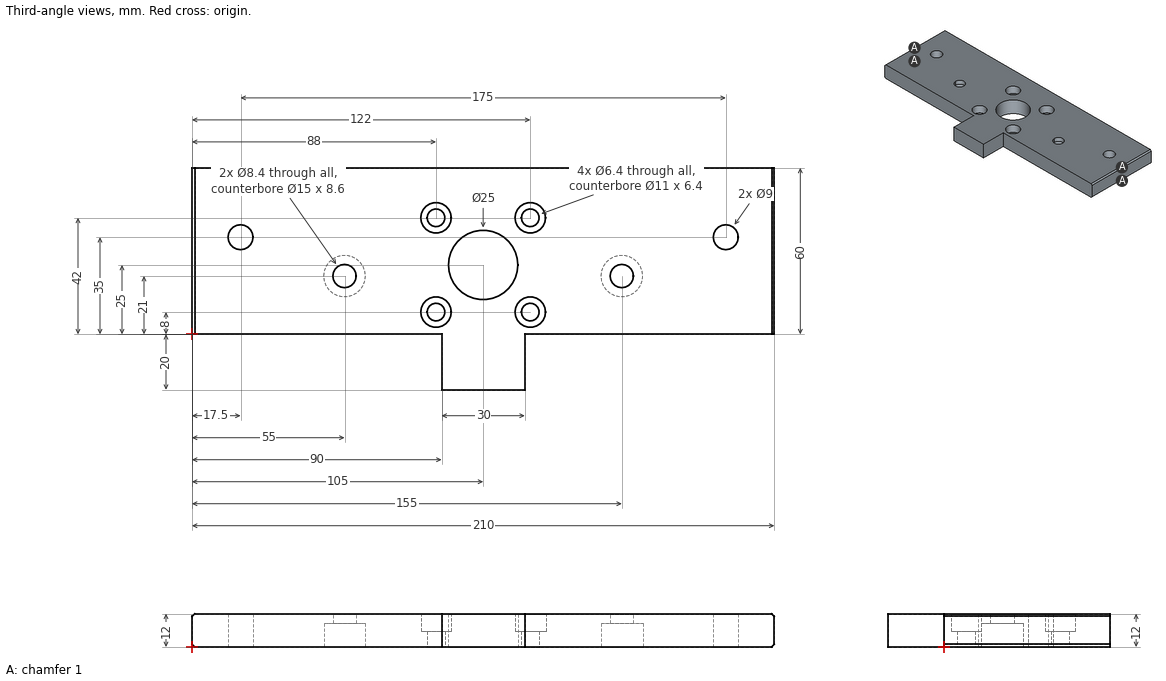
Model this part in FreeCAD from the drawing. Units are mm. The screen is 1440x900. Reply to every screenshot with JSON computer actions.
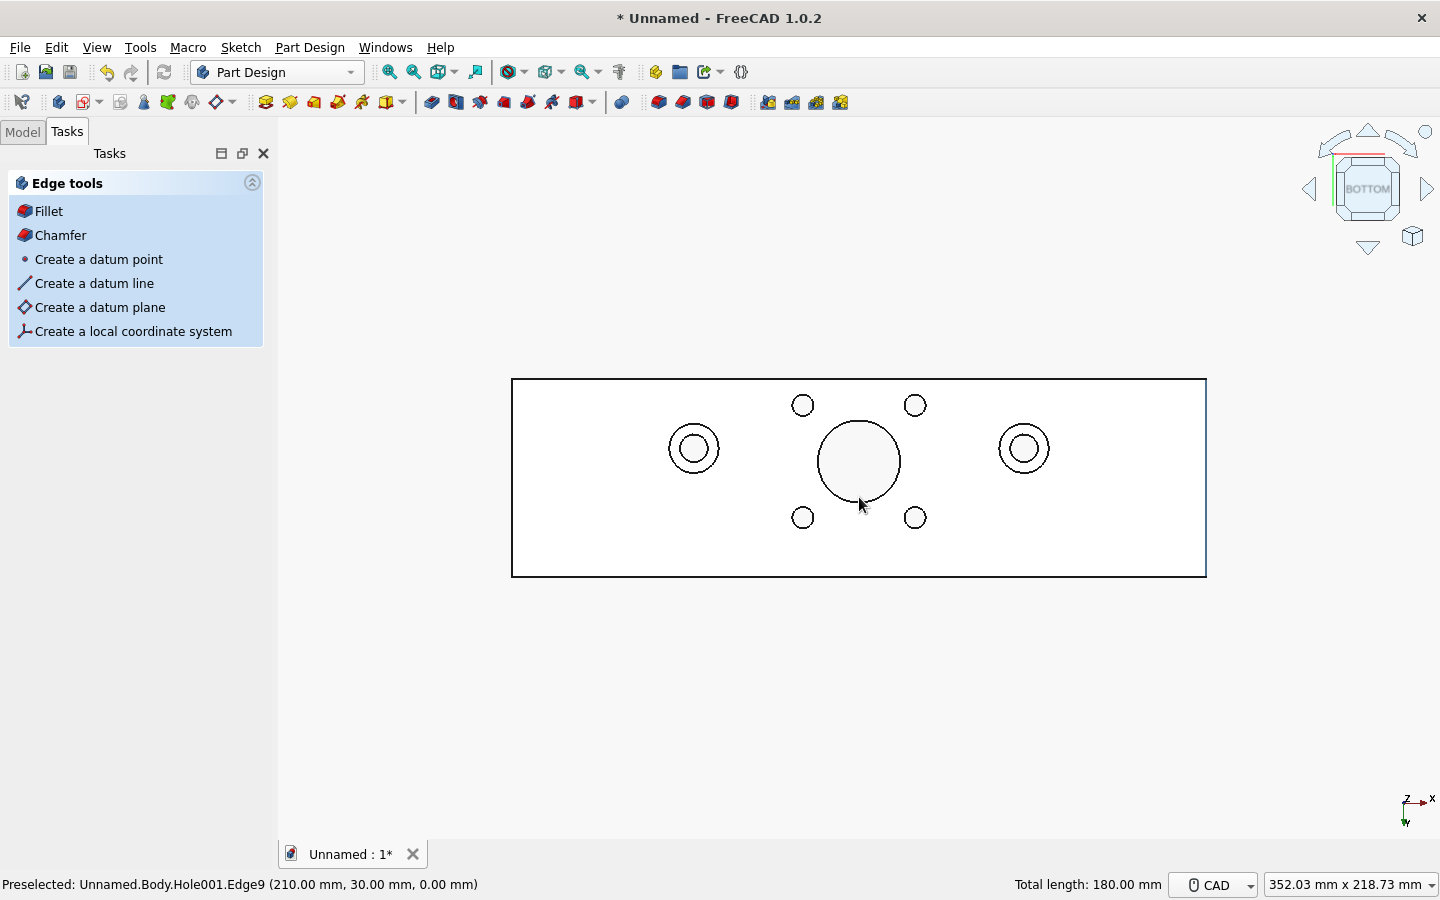
{"action": "left_click", "coordinate": [512, 477], "text": "ctrl"}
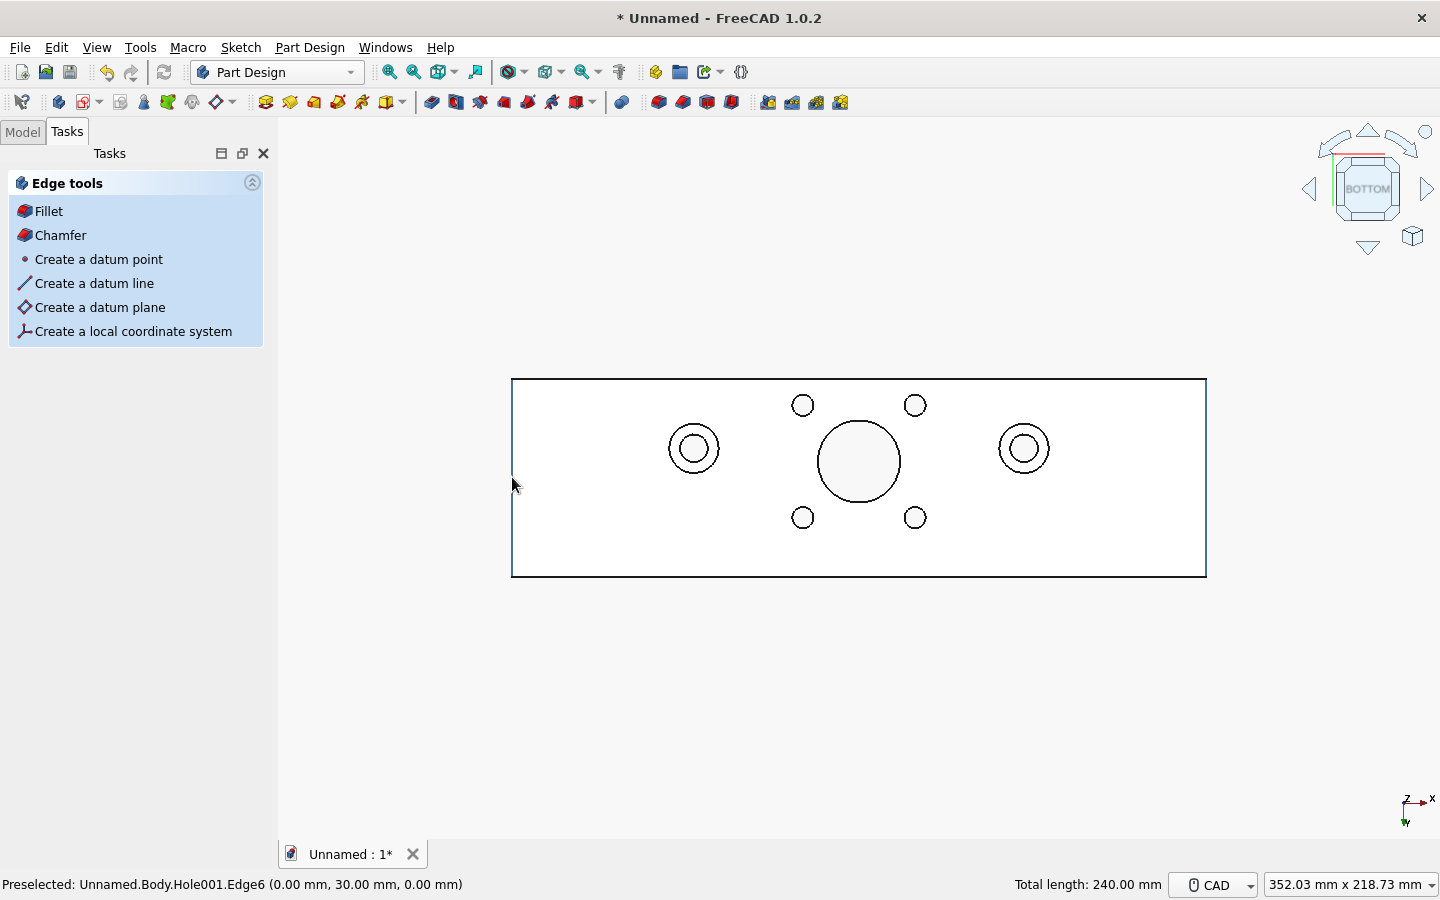
{"action": "left_click", "coordinate": [684, 102]}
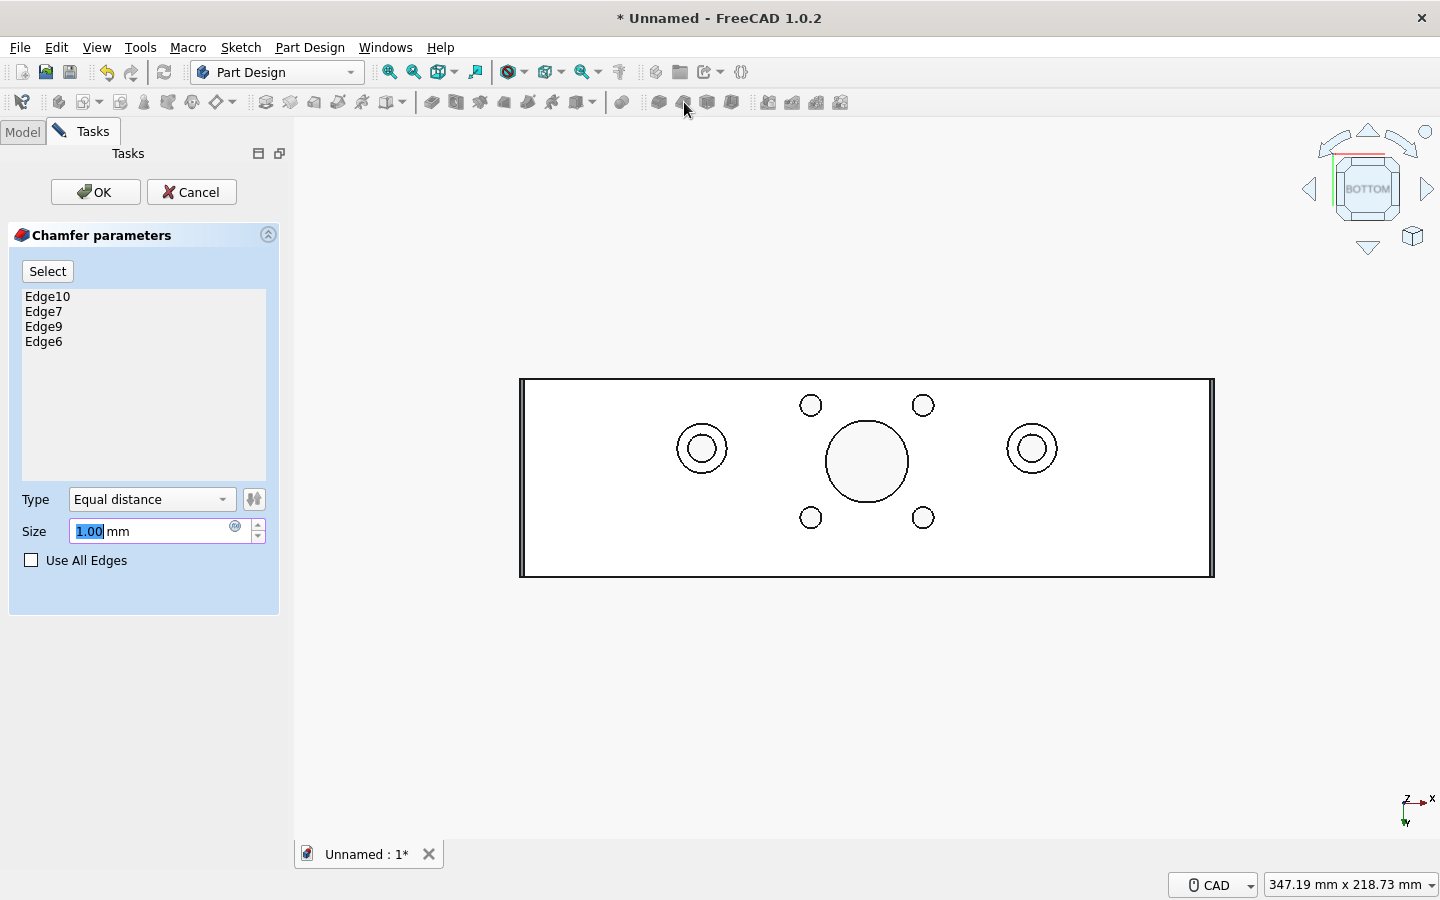
{"action": "type", "text": "1"}
{"action": "key", "text": "Tab"}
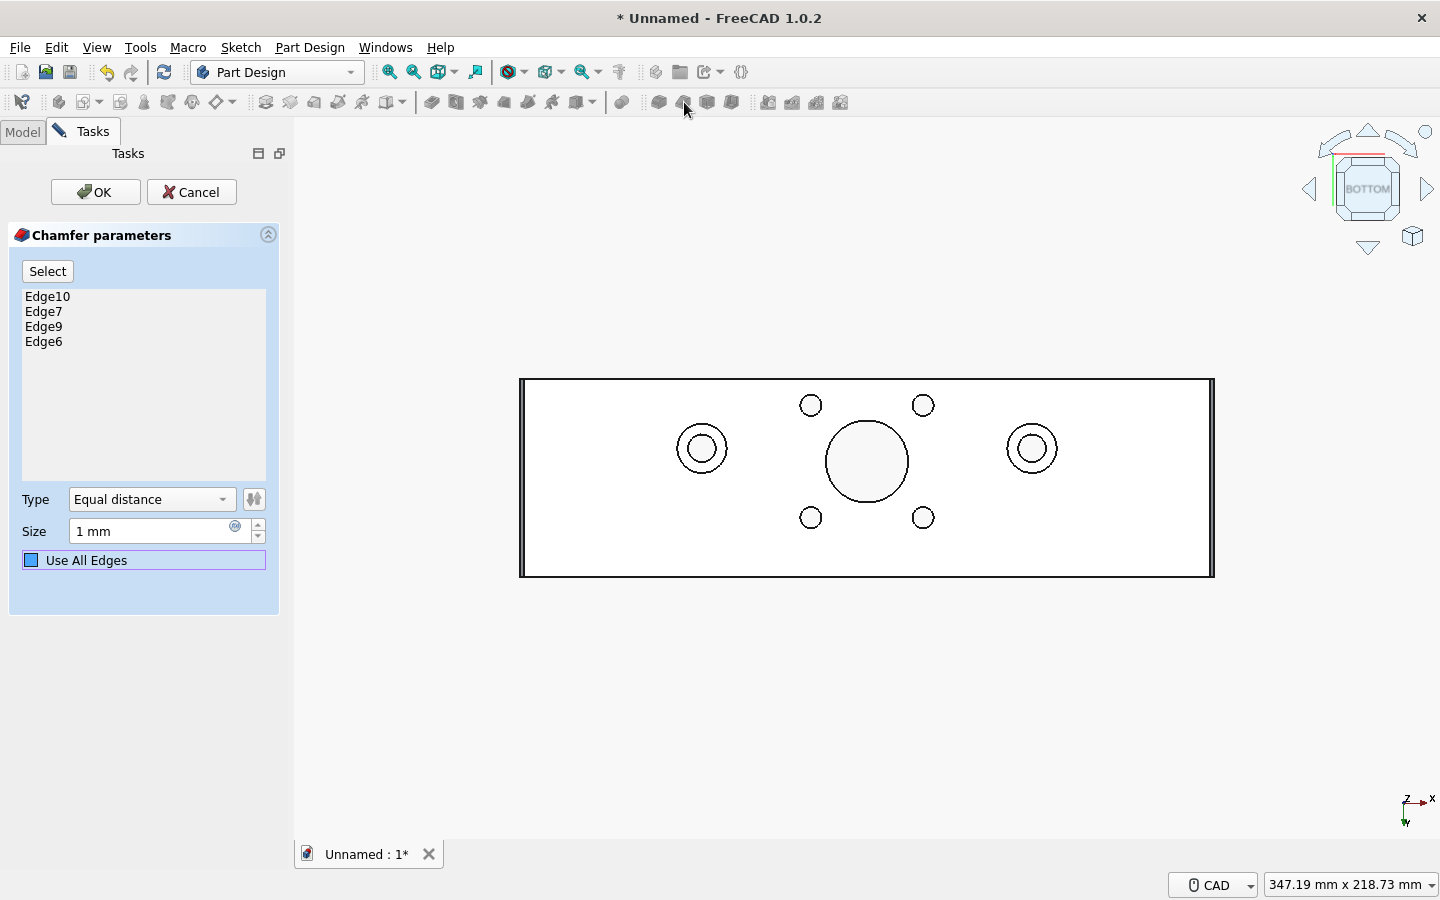
{"action": "left_click", "coordinate": [96, 192]}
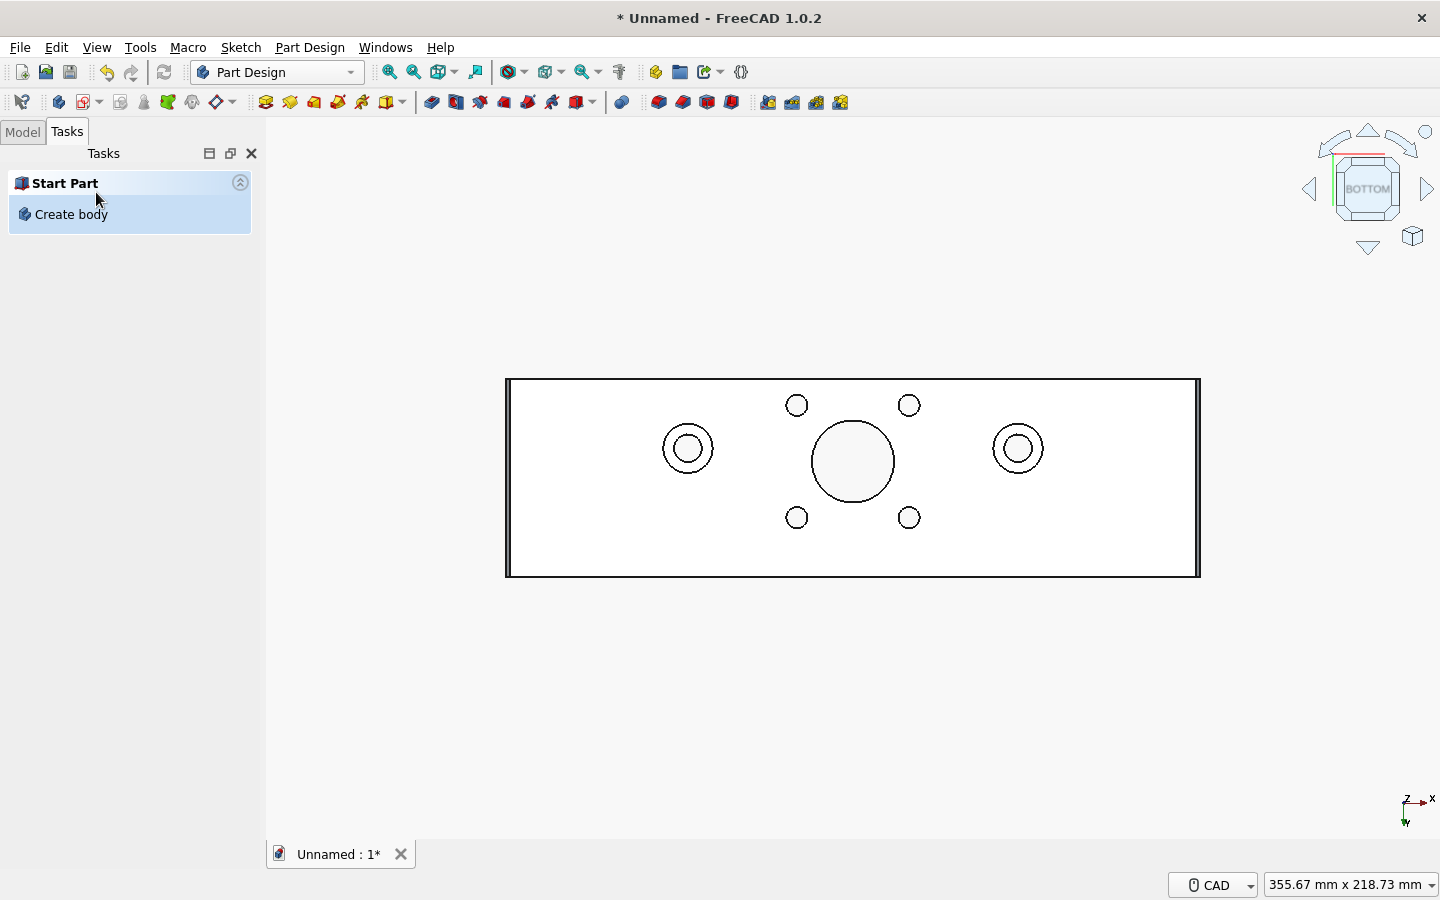
{"action": "left_click", "coordinate": [1147, 505]}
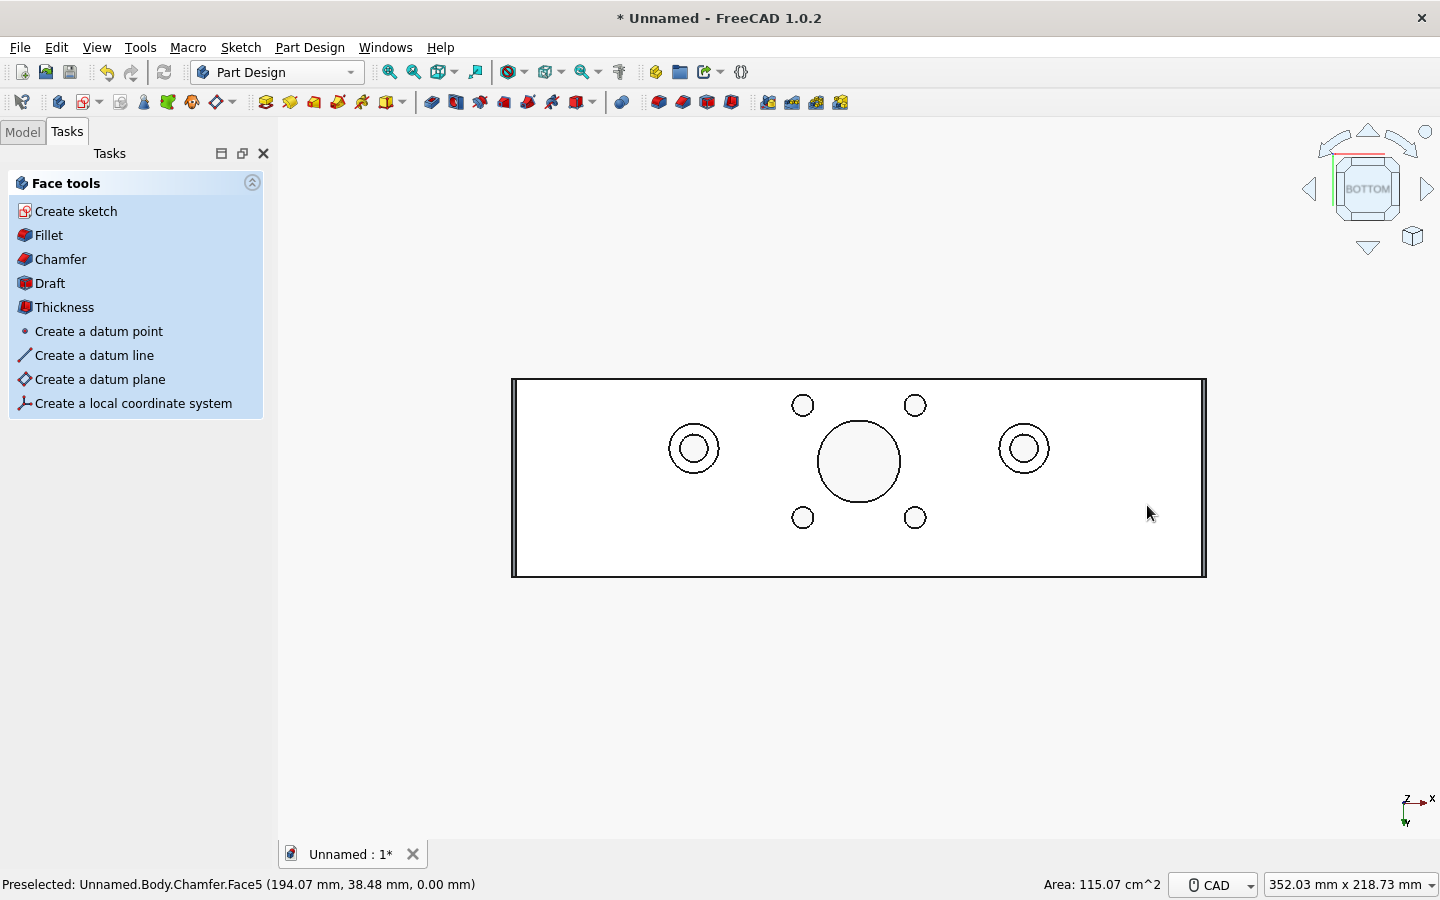
{"action": "left_click", "coordinate": [84, 102]}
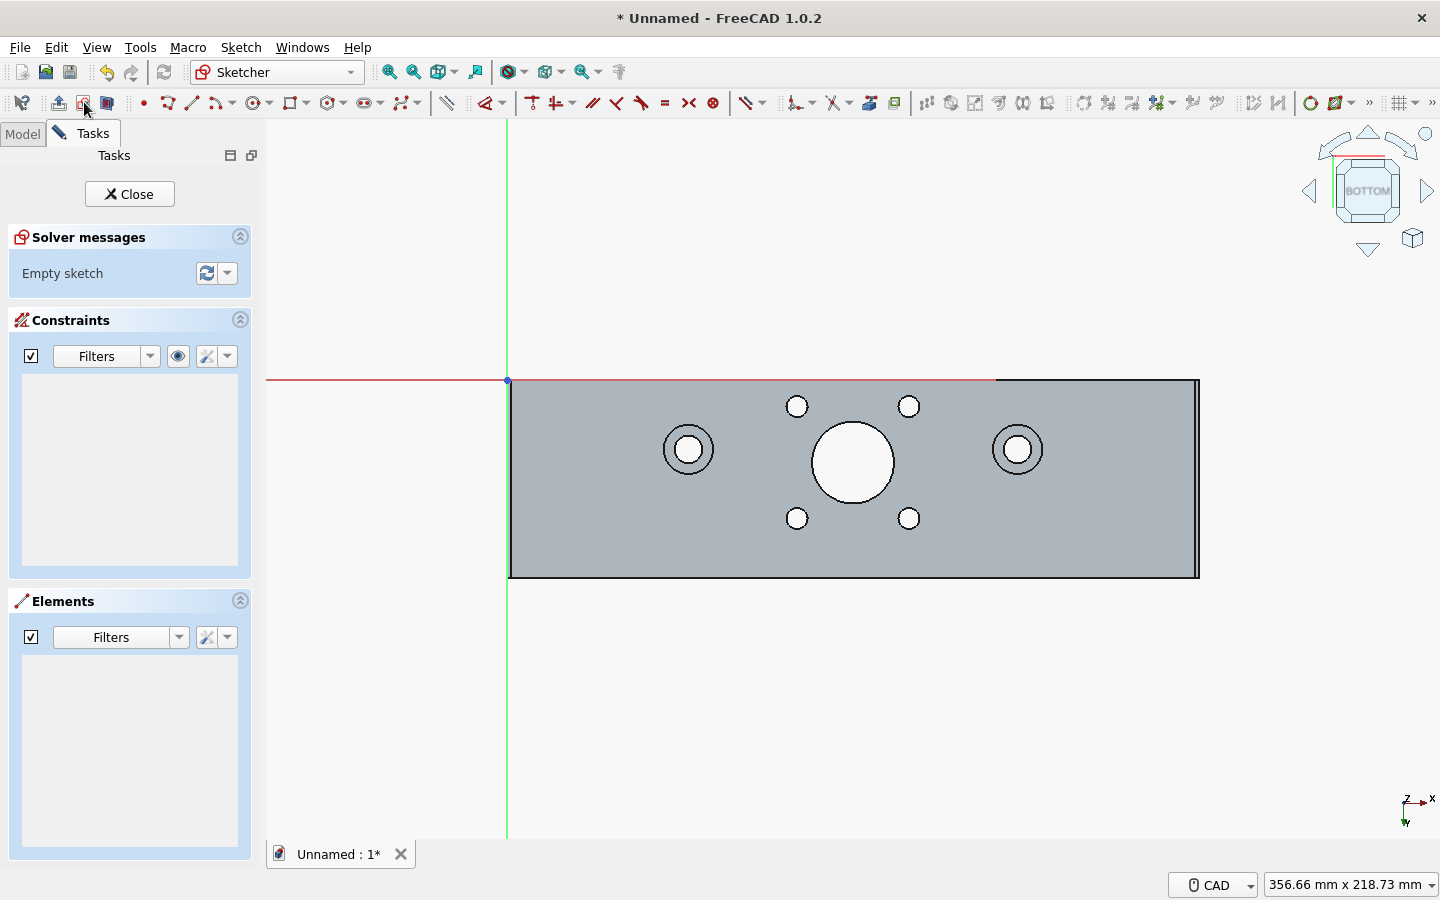
{"action": "key", "text": "g c"}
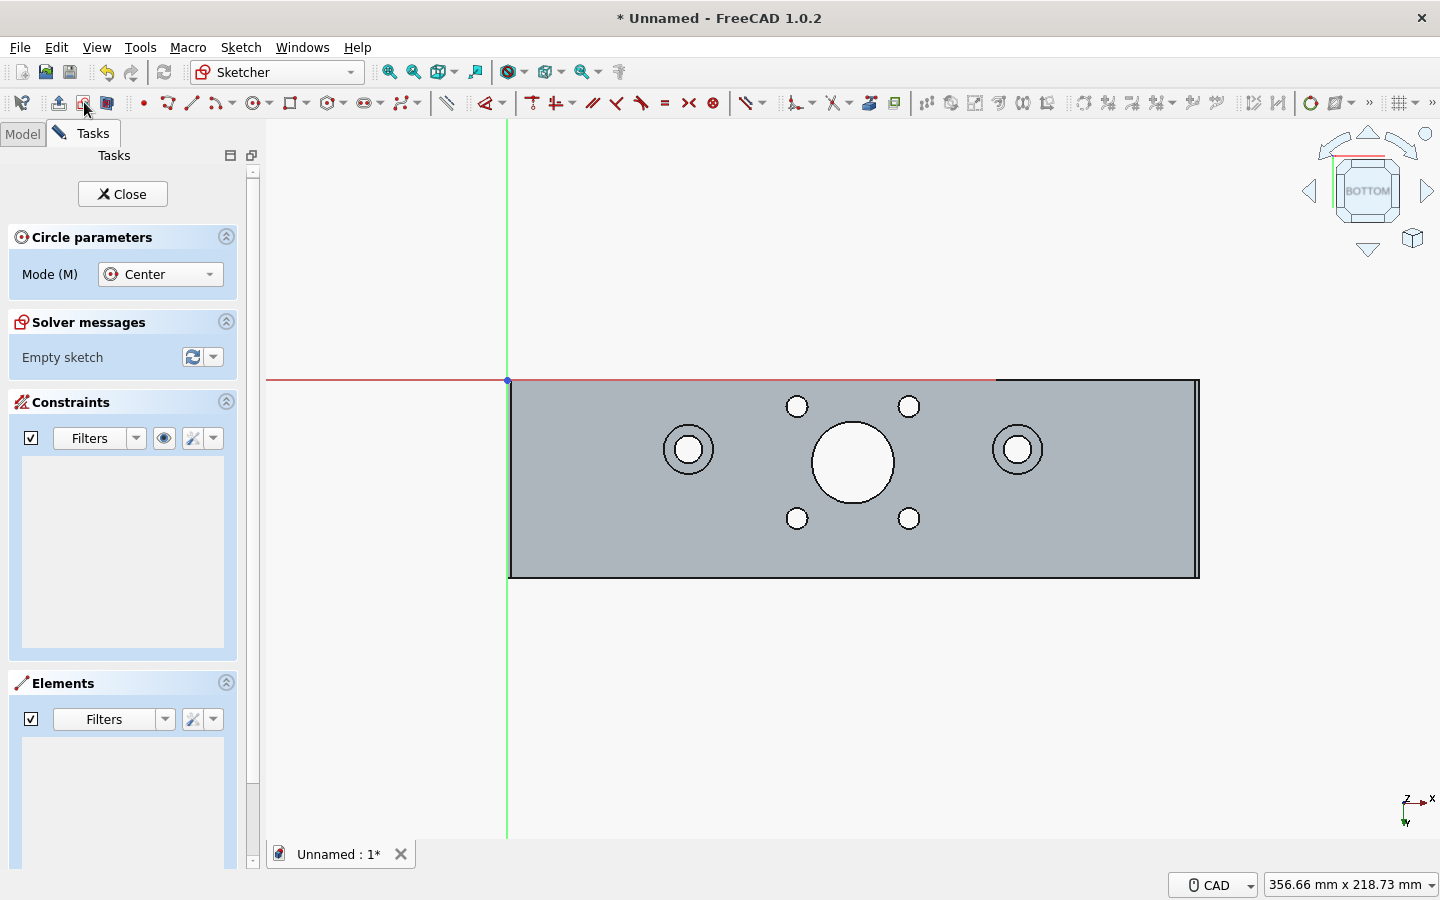
{"action": "scroll", "coordinate": [1141, 495], "scroll_direction": "up", "scroll_amount": 3}